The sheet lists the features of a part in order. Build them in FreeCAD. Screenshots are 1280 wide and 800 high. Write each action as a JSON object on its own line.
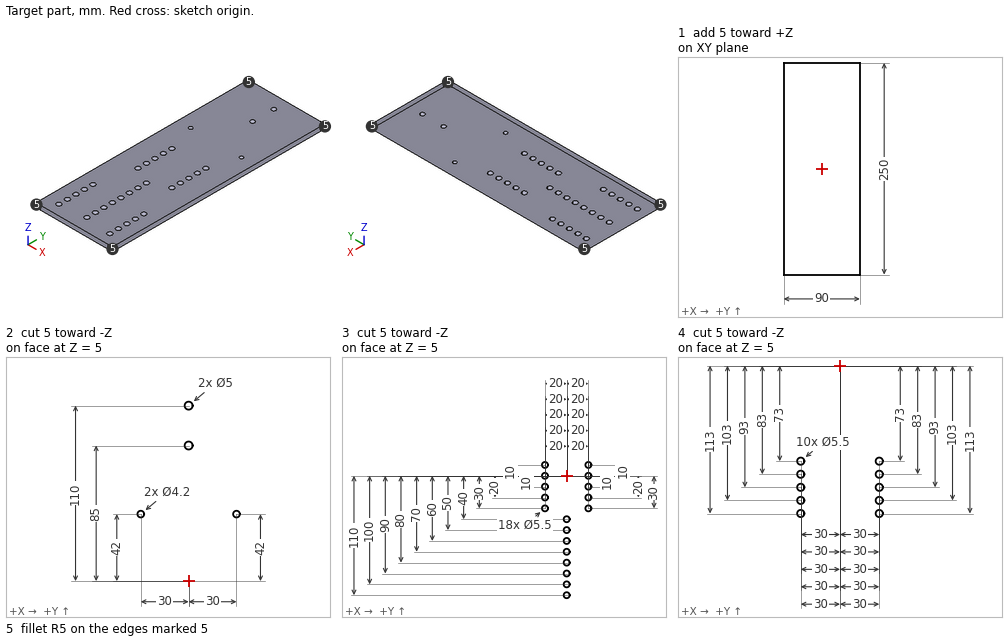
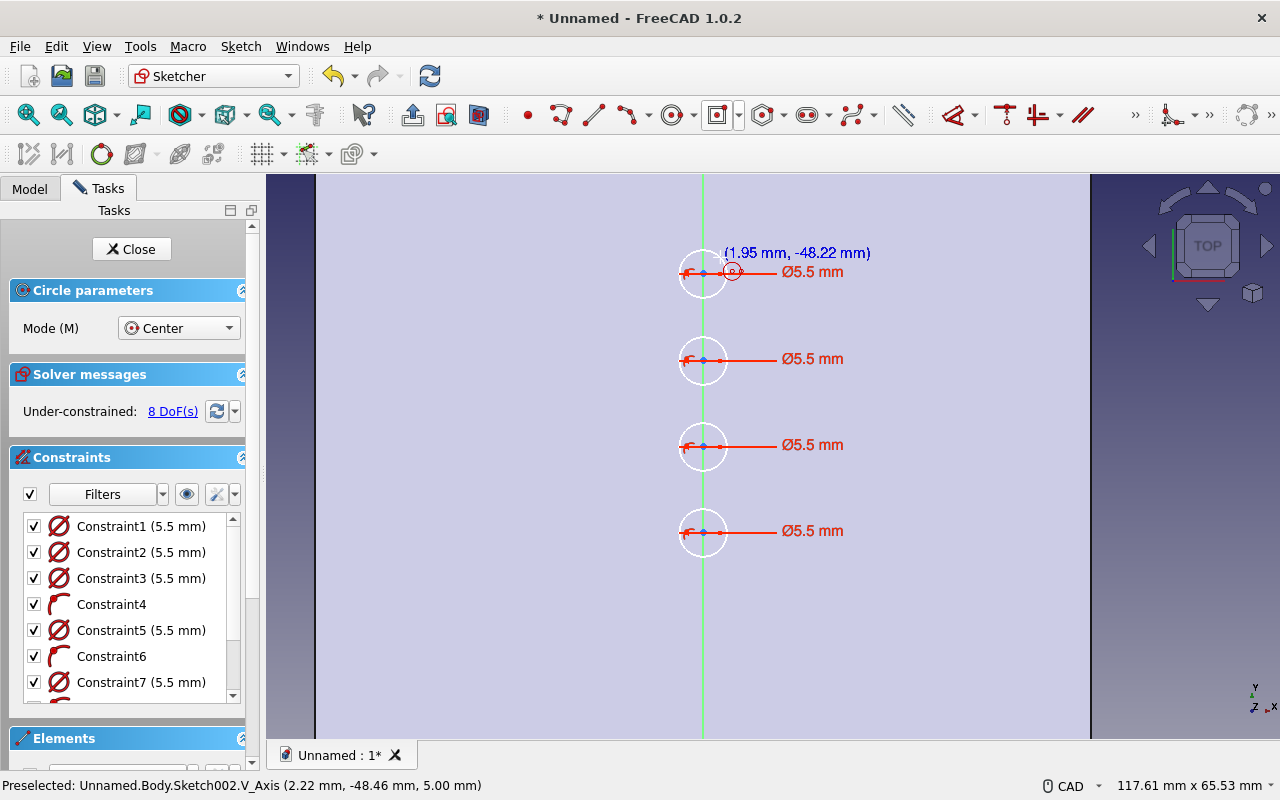
{"action": "scroll", "coordinate": [705, 535], "scroll_direction": "down", "scroll_amount": 6}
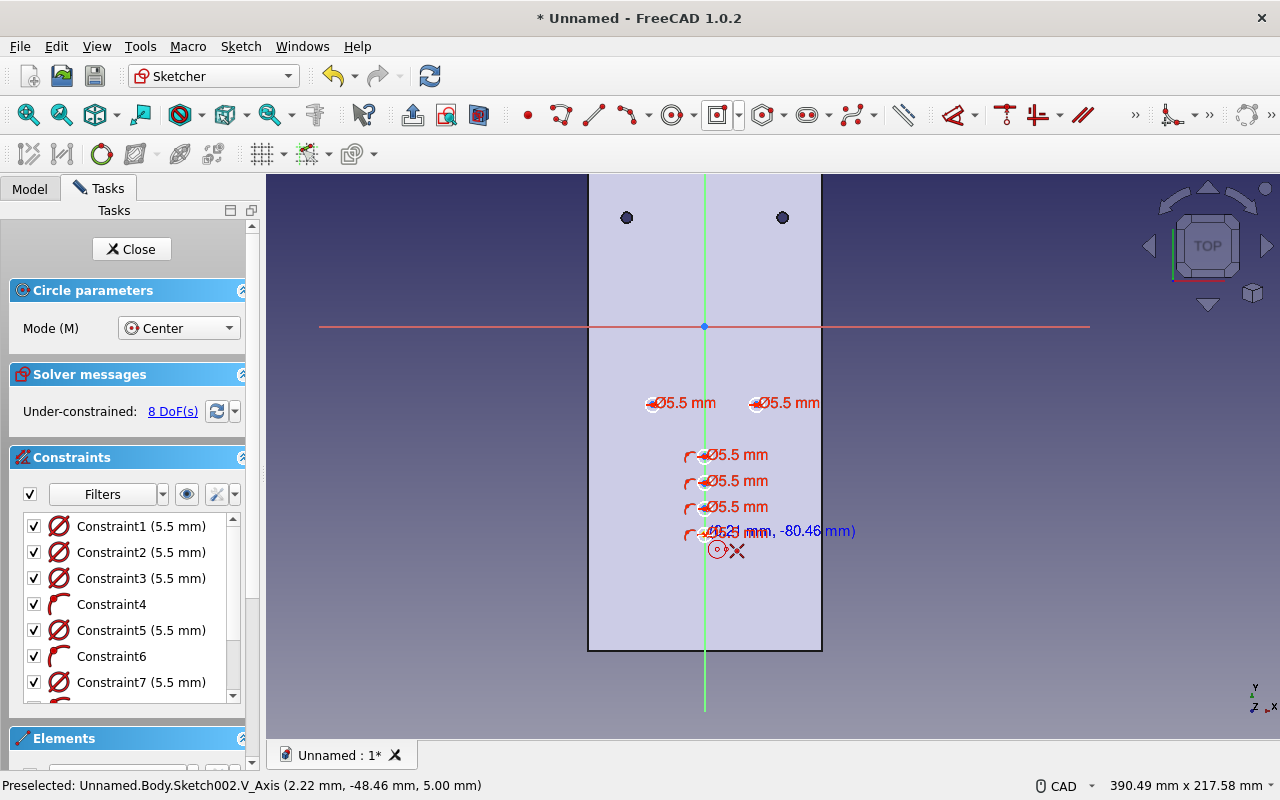
{"action": "scroll", "coordinate": [705, 431], "scroll_direction": "up", "scroll_amount": 6}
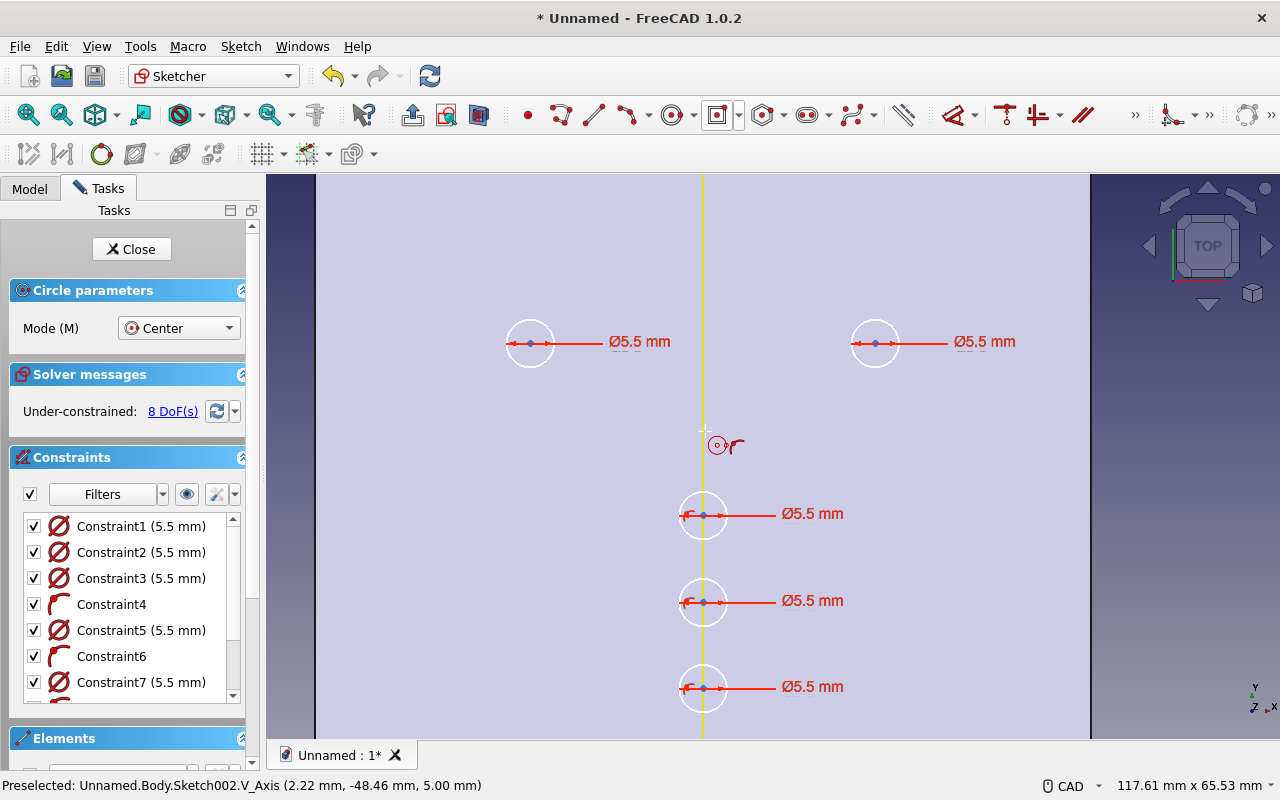
{"action": "left_click", "coordinate": [703, 429]}
{"action": "mouse_move", "coordinate": [720, 412]}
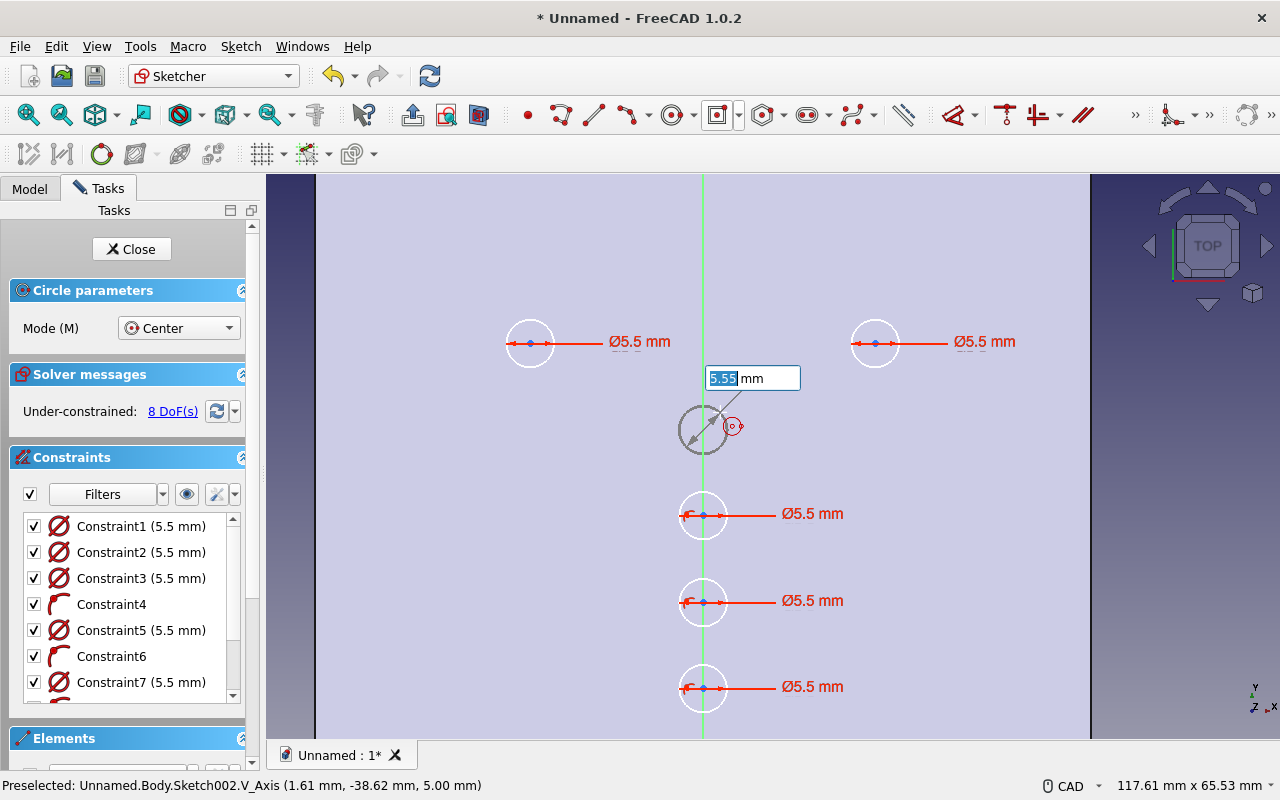
{"action": "type", "text": "5.5"}
{"action": "key", "text": "Return"}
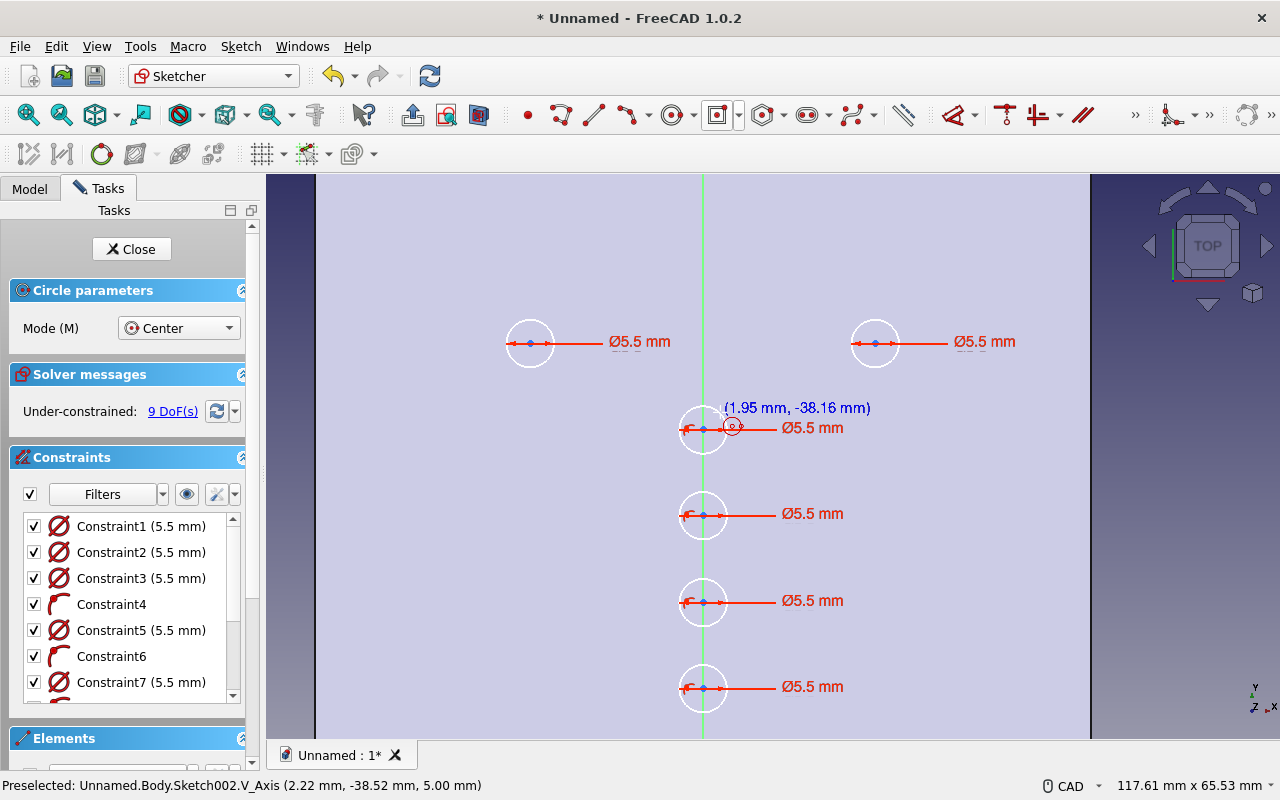
{"action": "scroll", "coordinate": [705, 431], "scroll_direction": "down", "scroll_amount": 6}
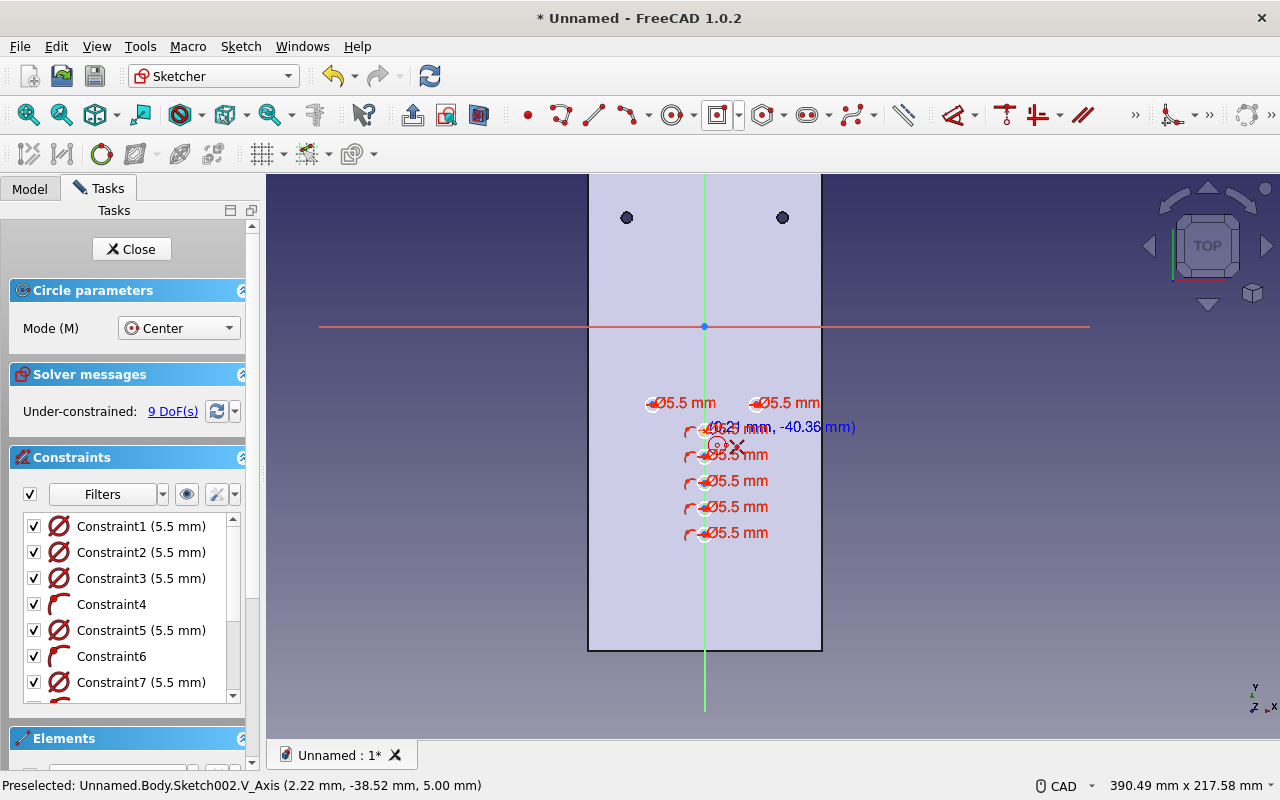
{"action": "scroll", "coordinate": [705, 561], "scroll_direction": "up", "scroll_amount": 6}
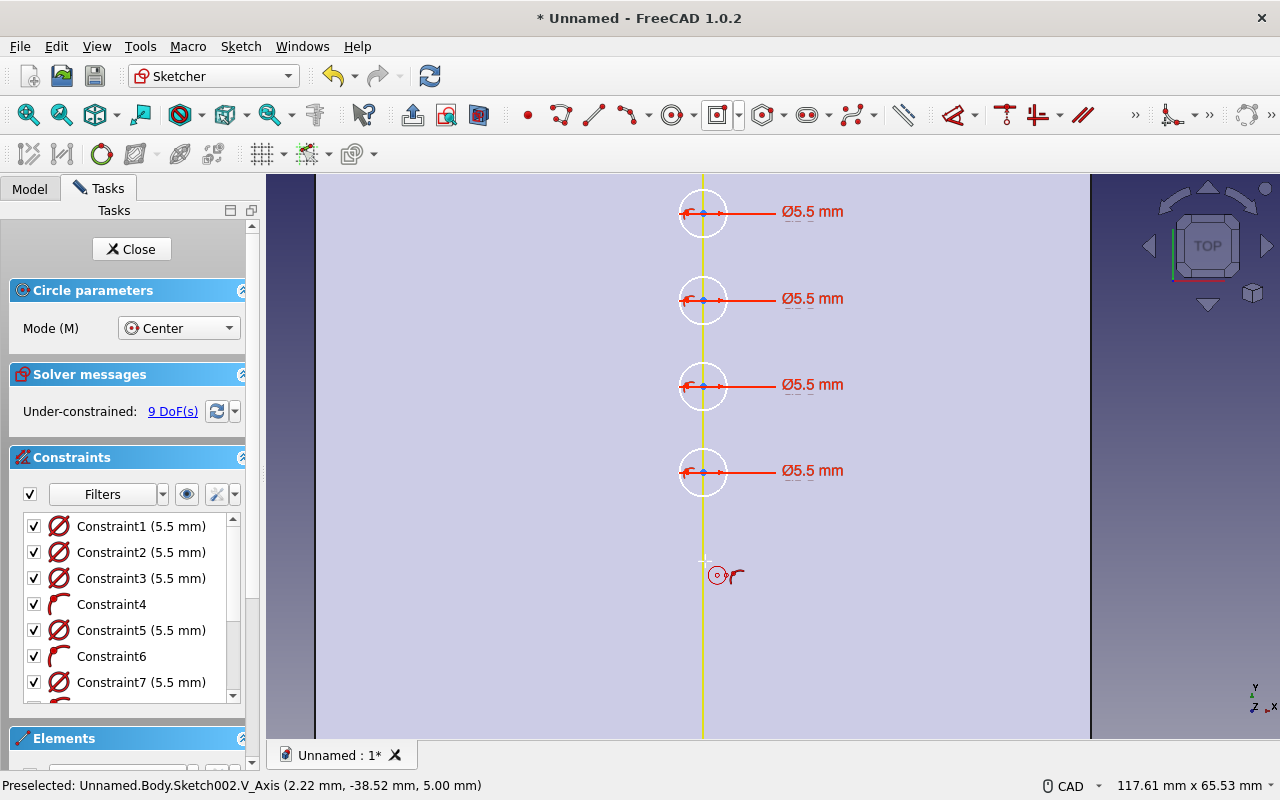
{"action": "left_click", "coordinate": [703, 558]}
{"action": "mouse_move", "coordinate": [720, 541]}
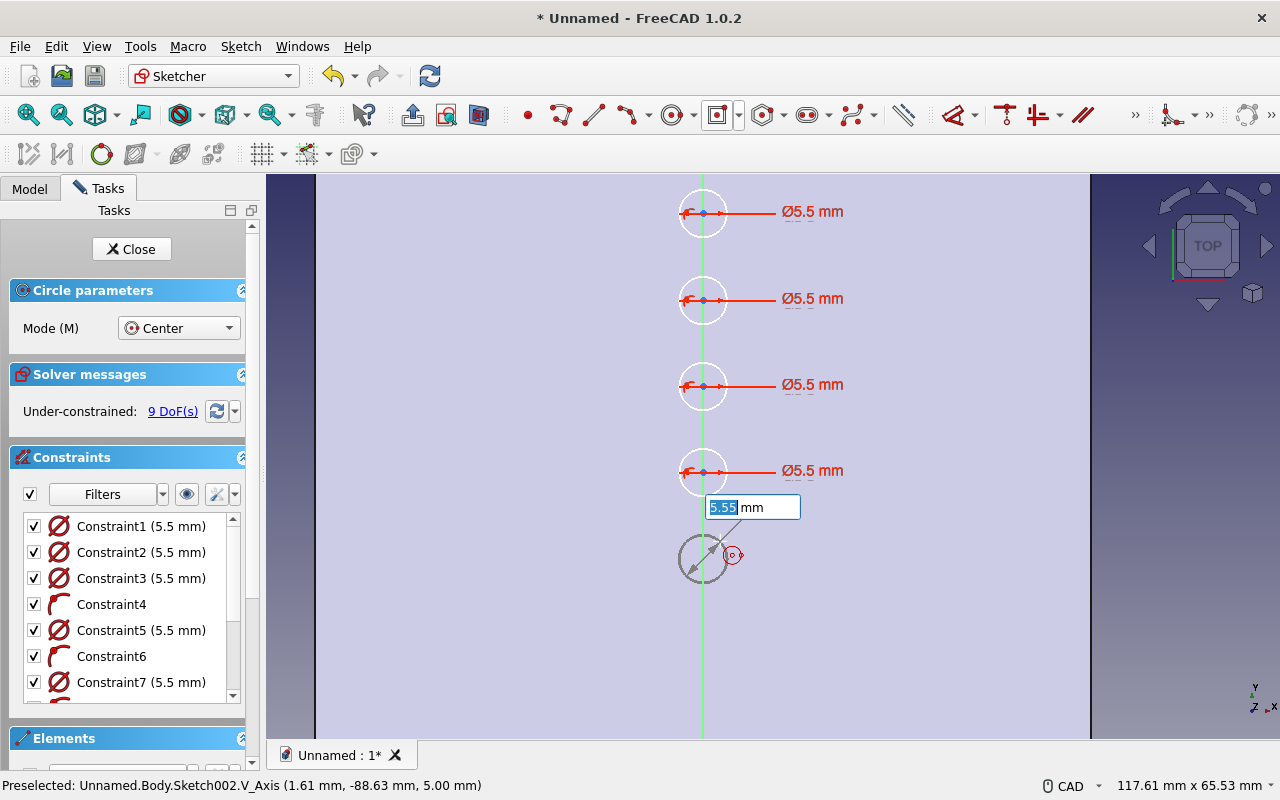
{"action": "type", "text": "5.5"}
{"action": "key", "text": "Return"}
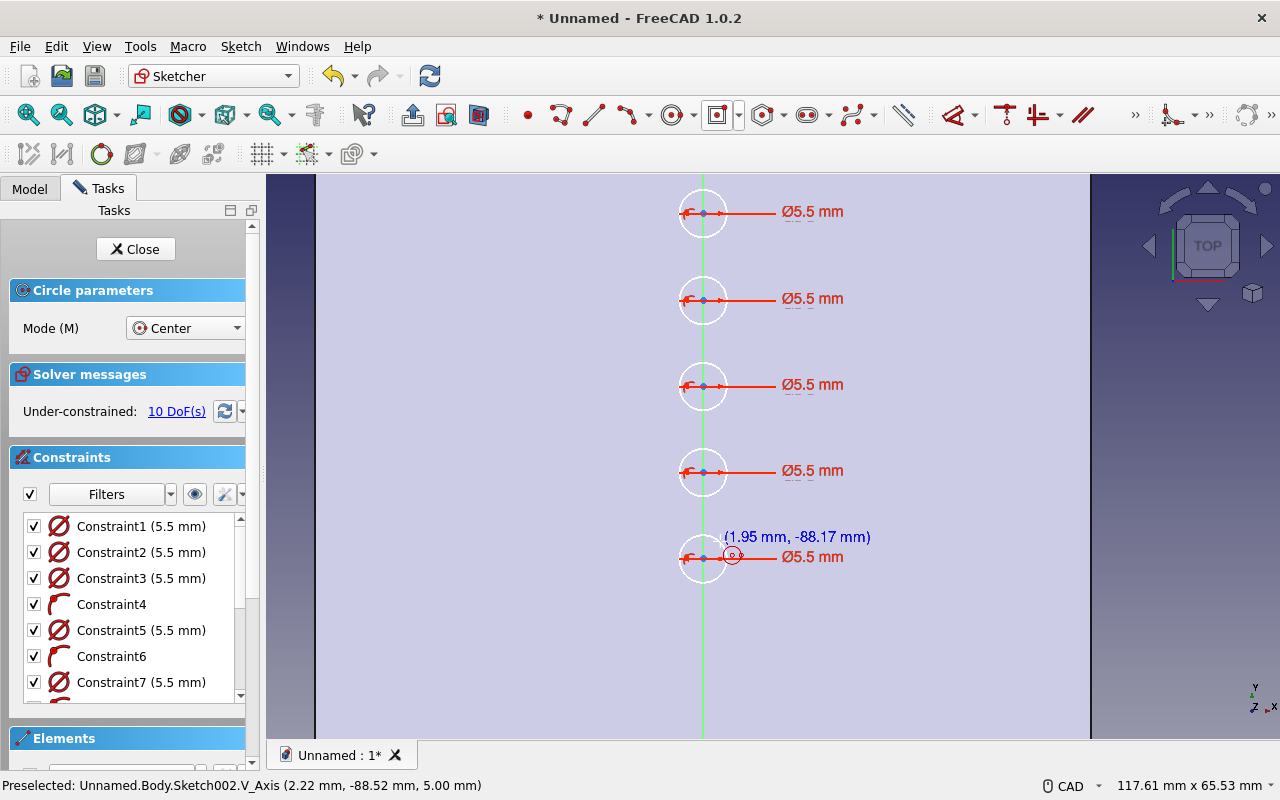
{"action": "left_click", "coordinate": [703, 644]}
{"action": "mouse_move", "coordinate": [720, 627]}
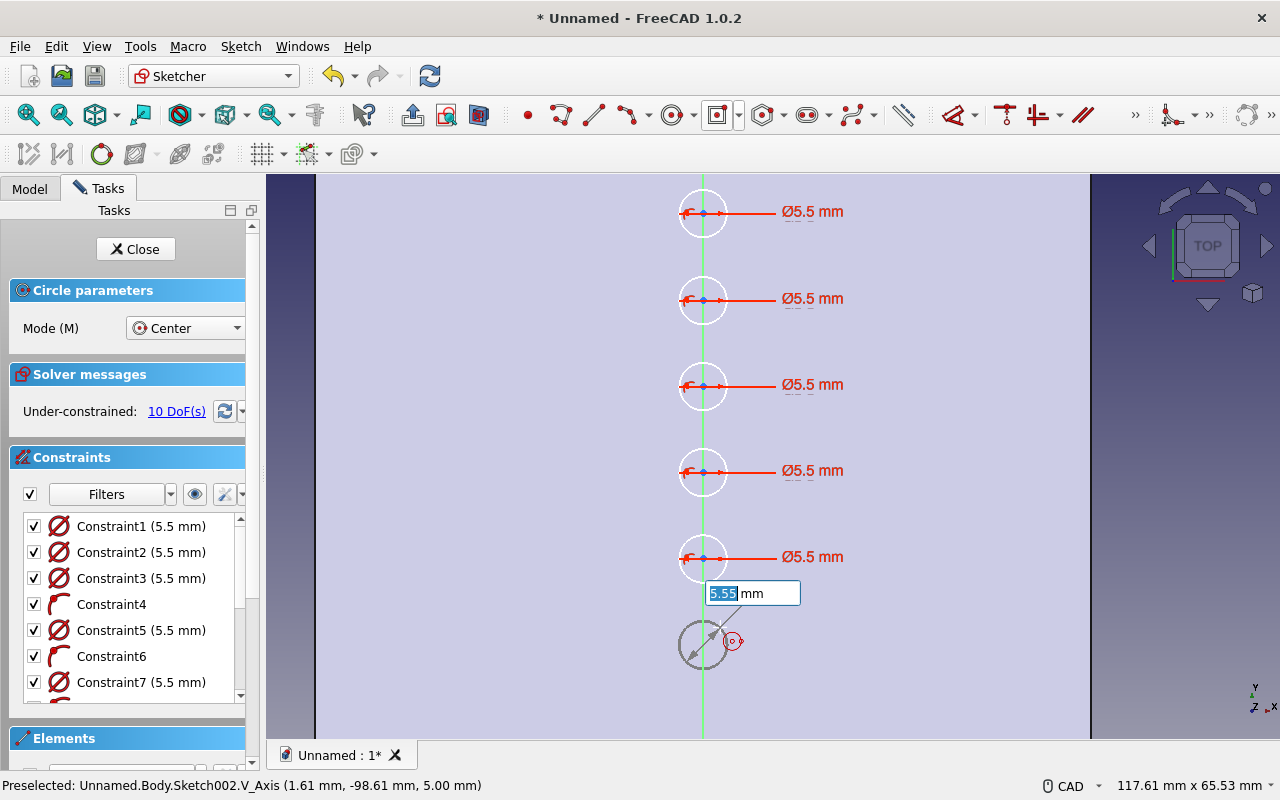
{"action": "type", "text": "5.5"}
{"action": "key", "text": "Return"}